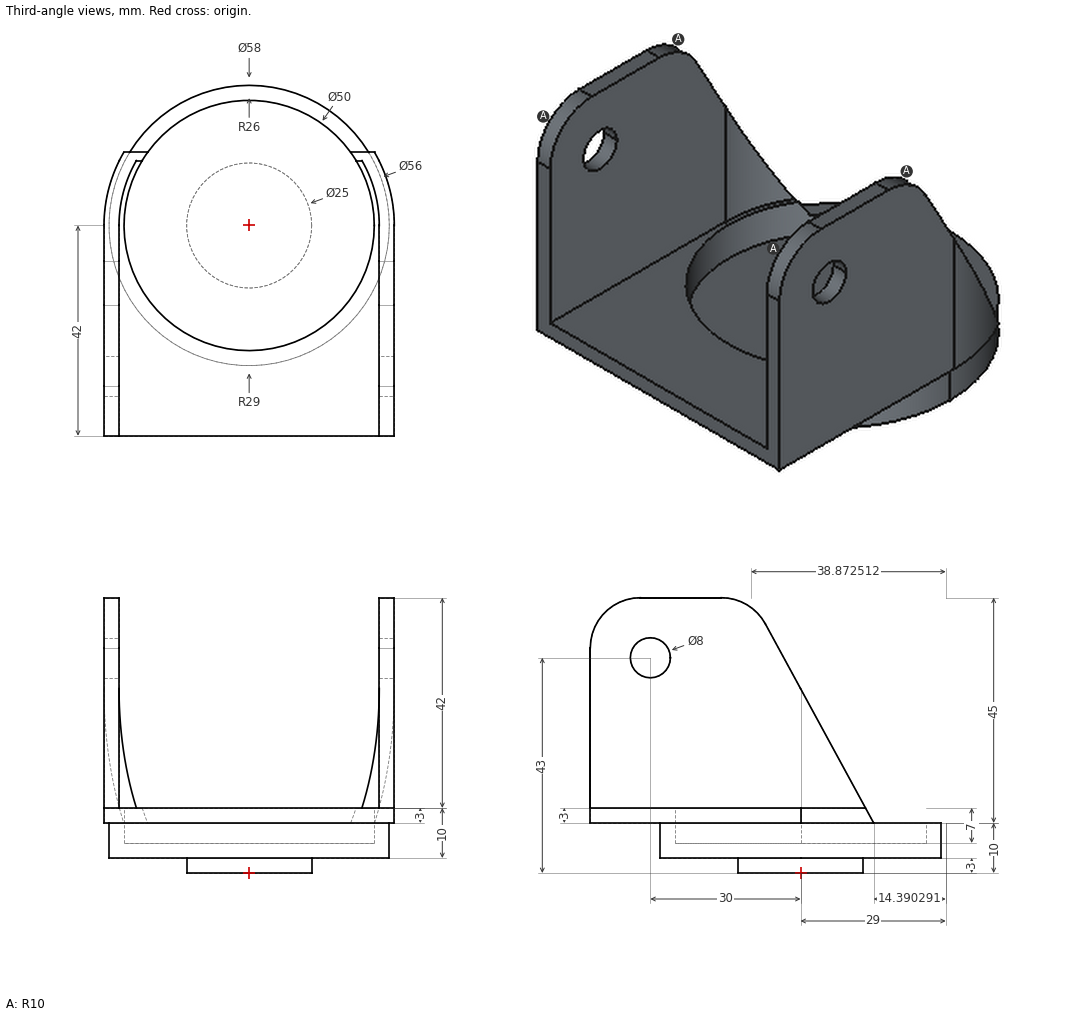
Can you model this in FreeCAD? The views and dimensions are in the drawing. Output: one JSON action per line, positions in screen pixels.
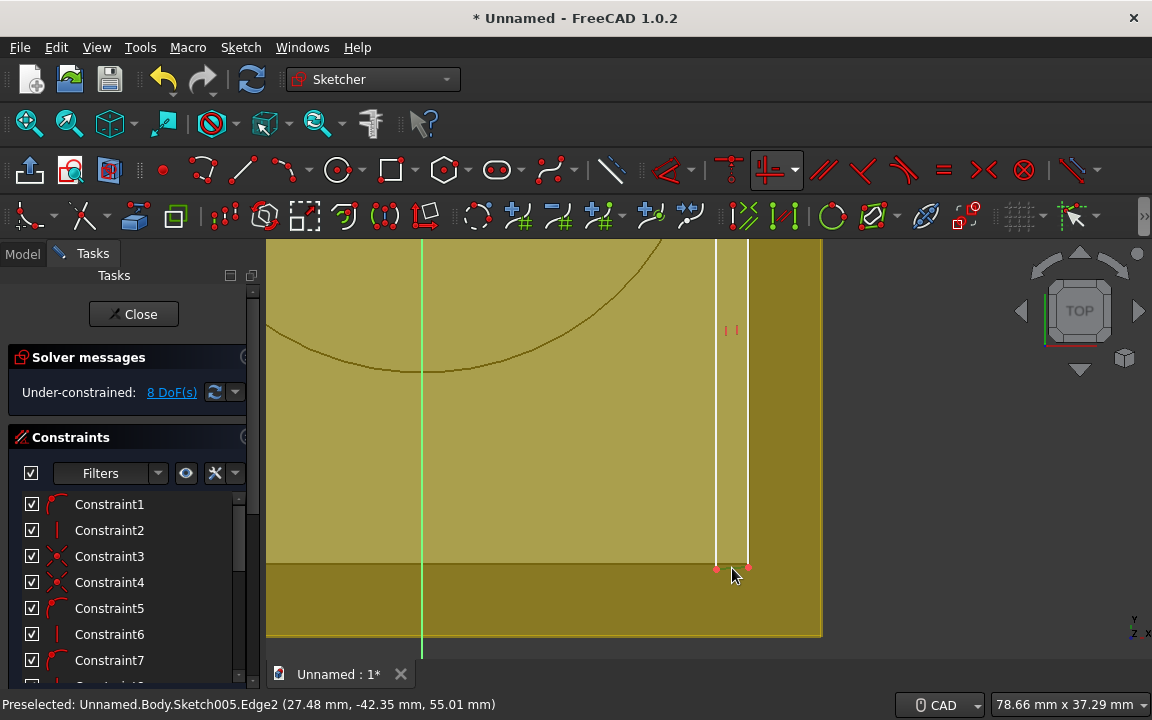
{"action": "key", "text": "h"}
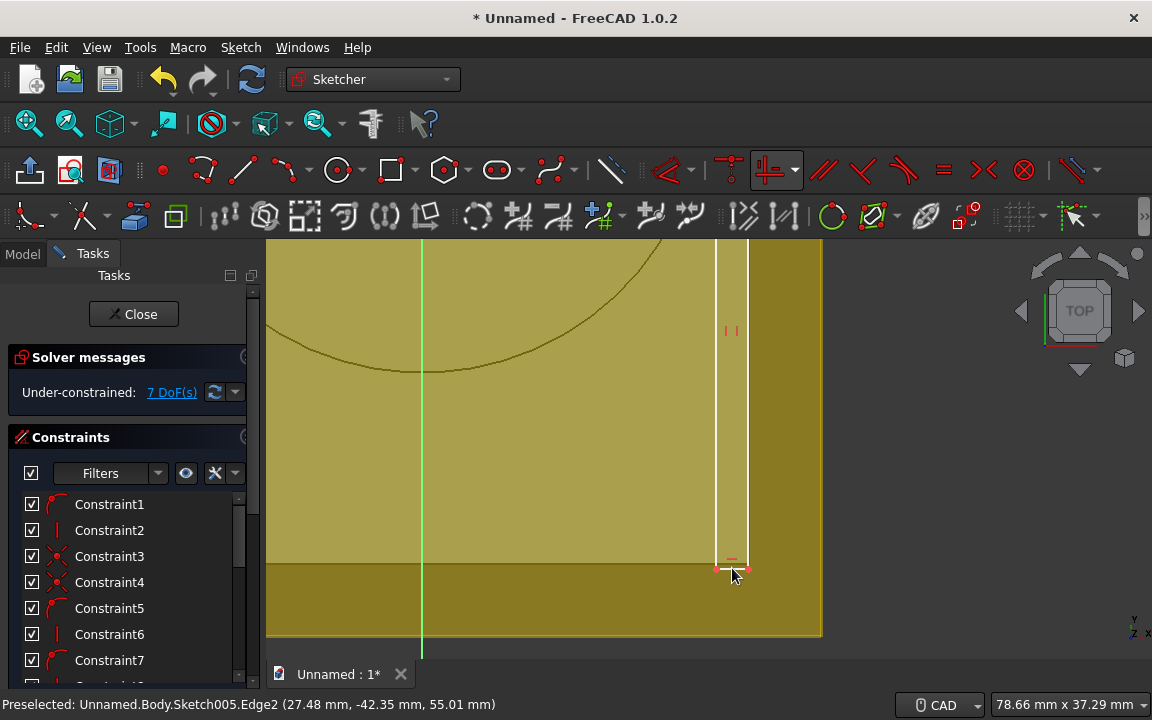
{"action": "scroll", "coordinate": [735, 572], "scroll_direction": "down", "scroll_amount": 6}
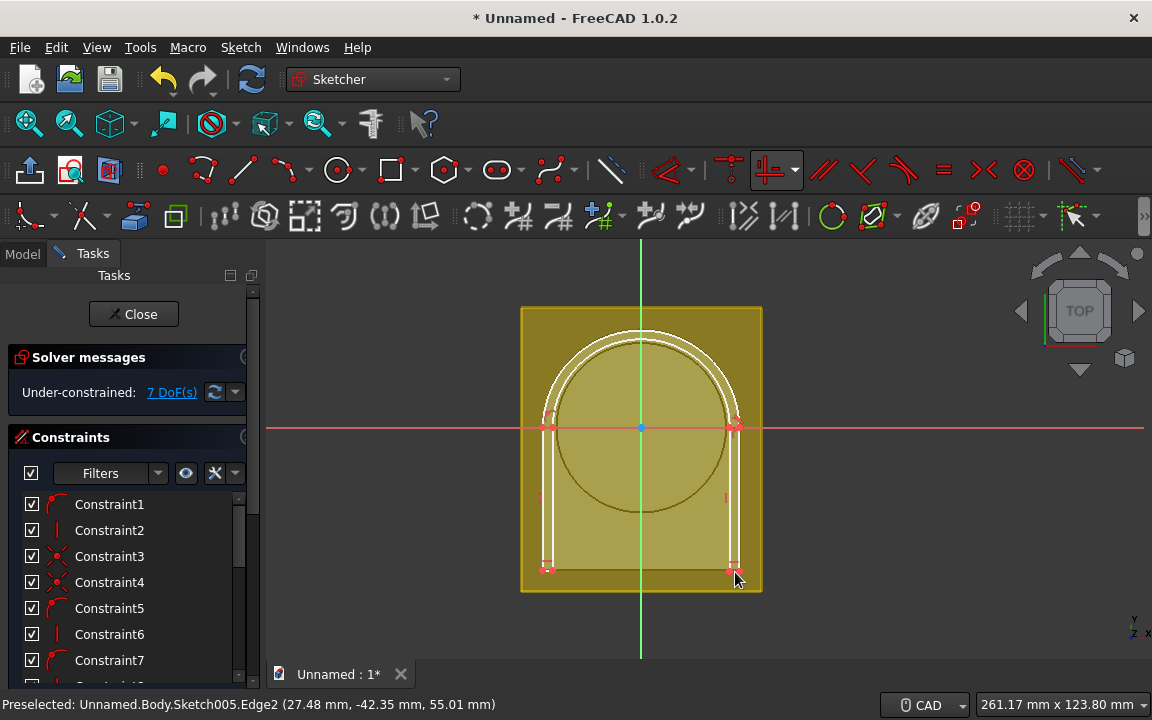
{"action": "scroll", "coordinate": [699, 349], "scroll_direction": "up", "scroll_amount": 3}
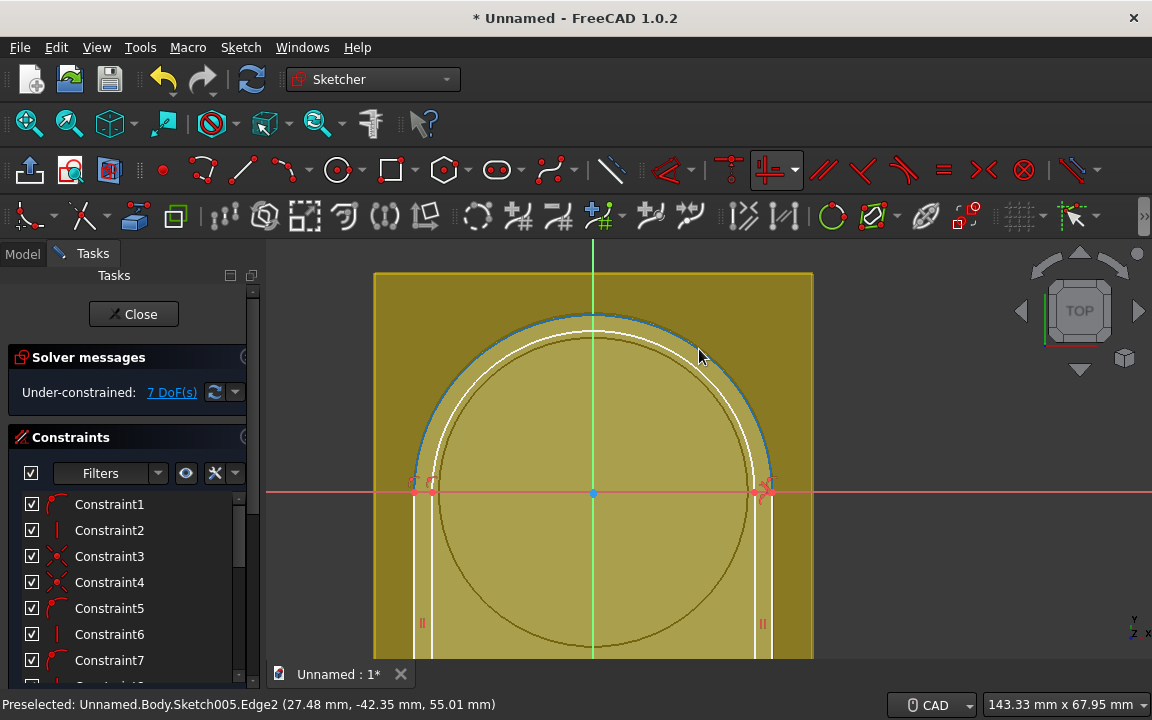
{"action": "left_click", "coordinate": [698, 349]}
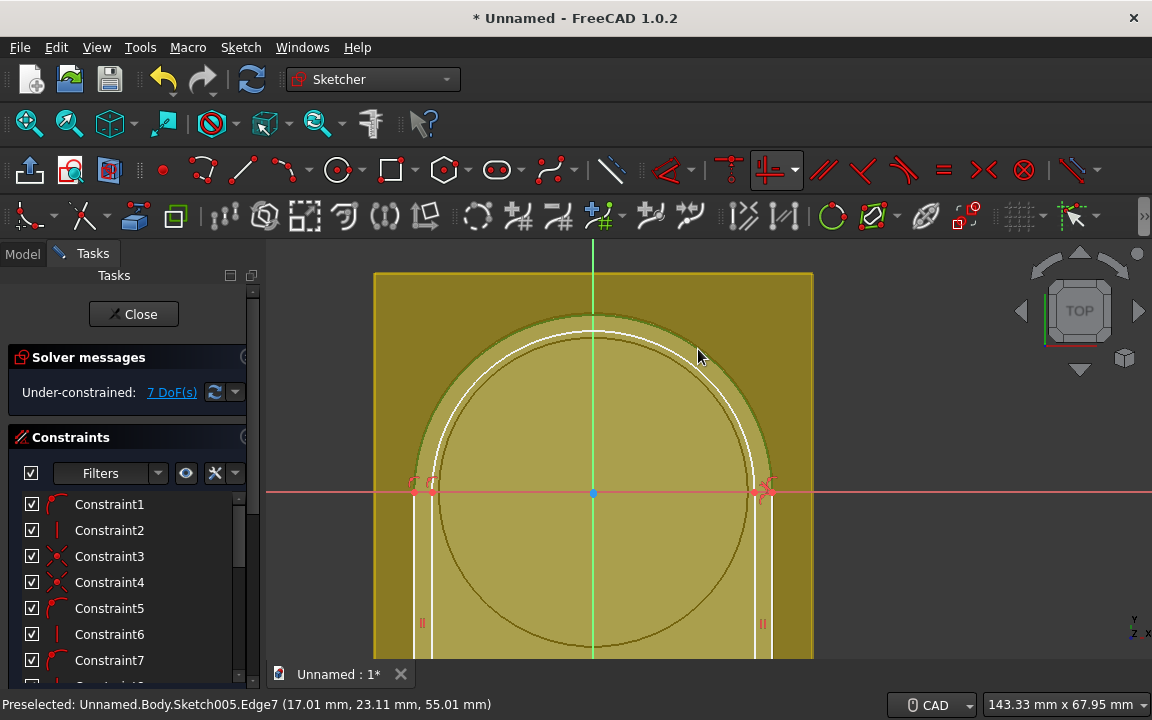
{"action": "left_click", "coordinate": [688, 362]}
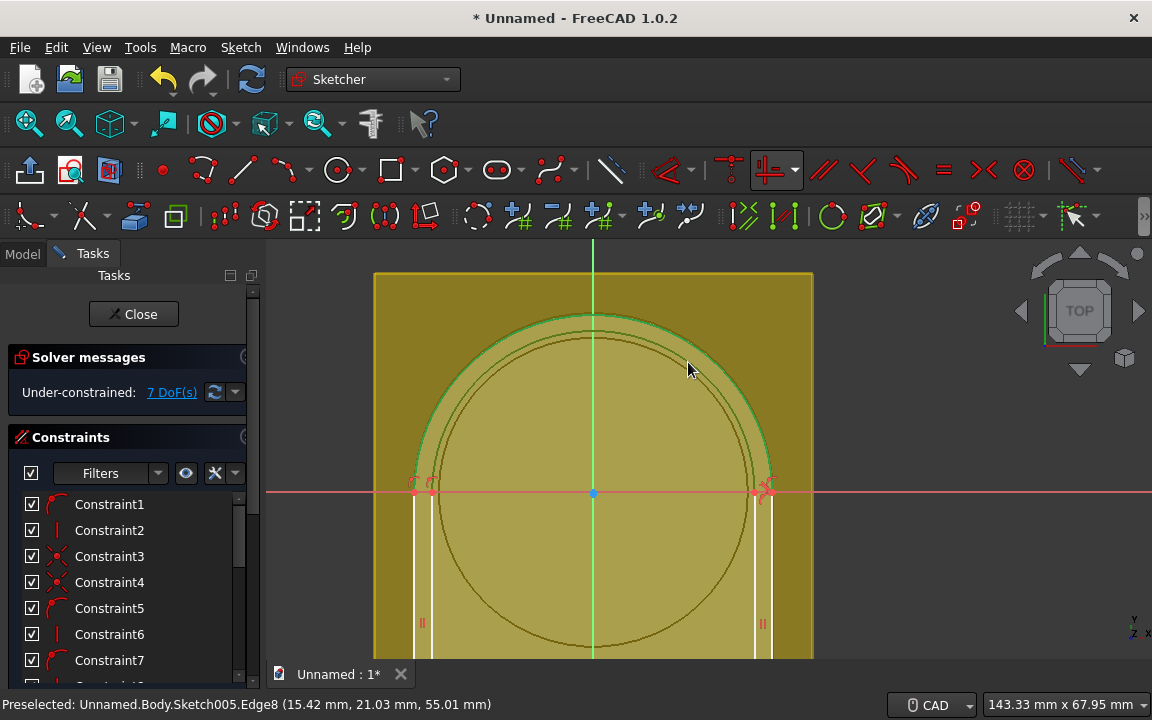
{"action": "left_click", "coordinate": [730, 170]}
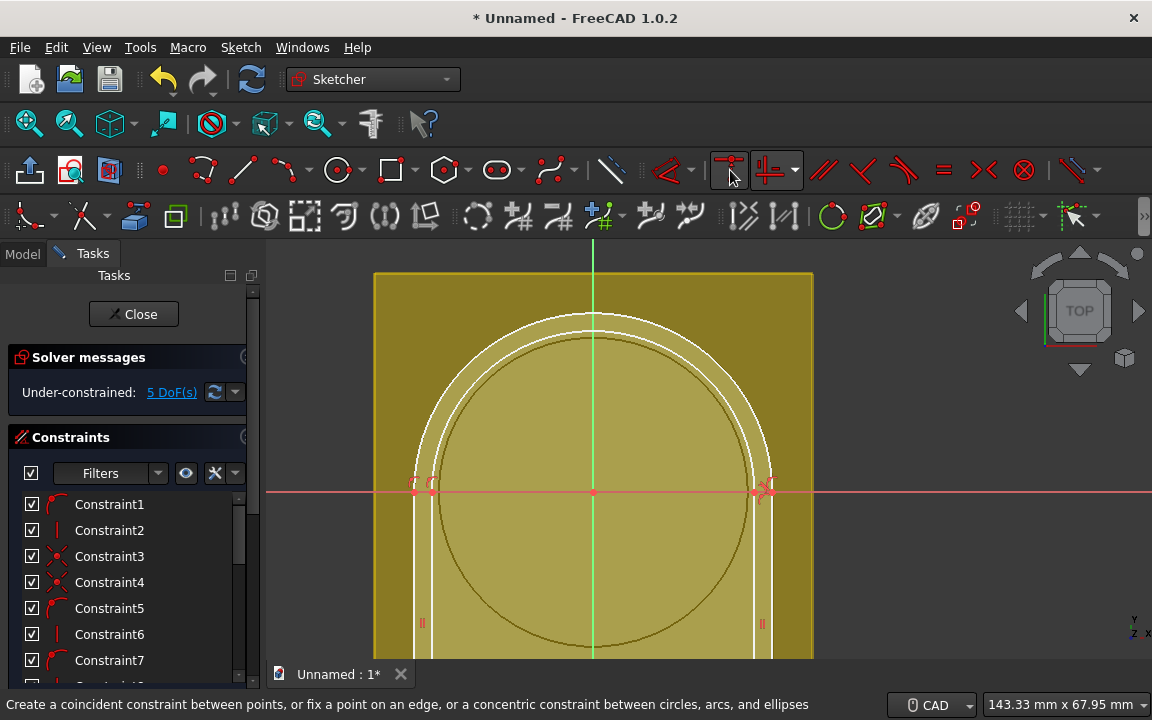
{"action": "left_click", "coordinate": [593, 492]}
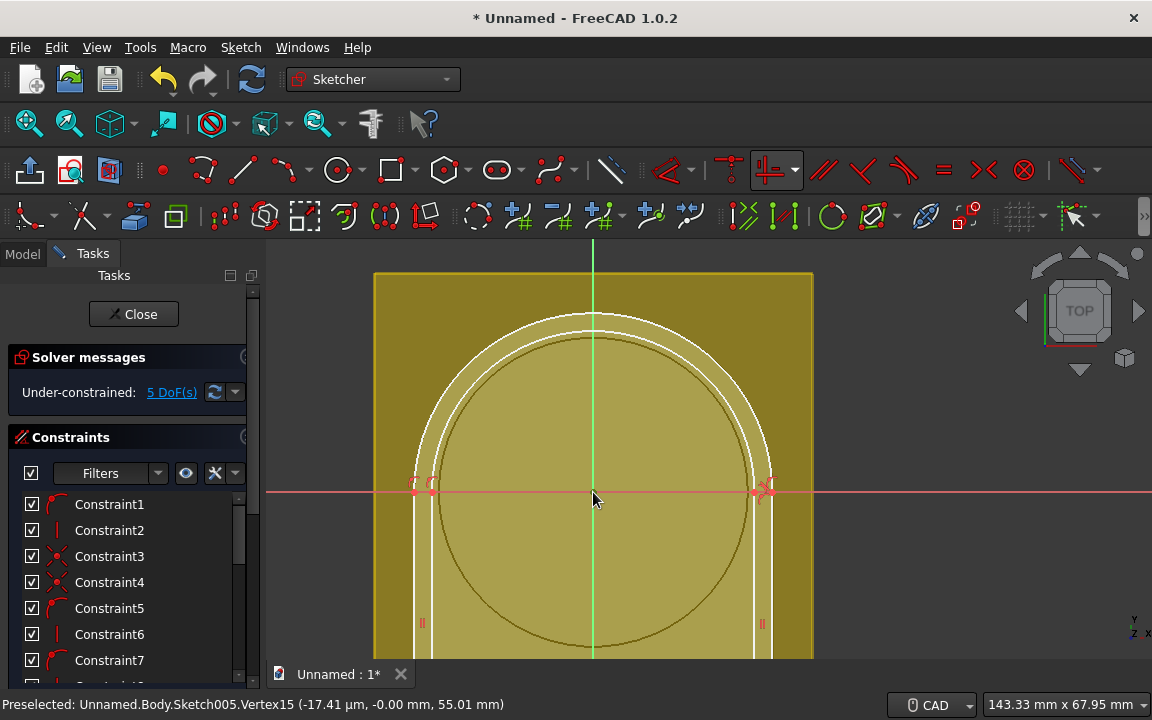
{"action": "left_click", "coordinate": [593, 605]}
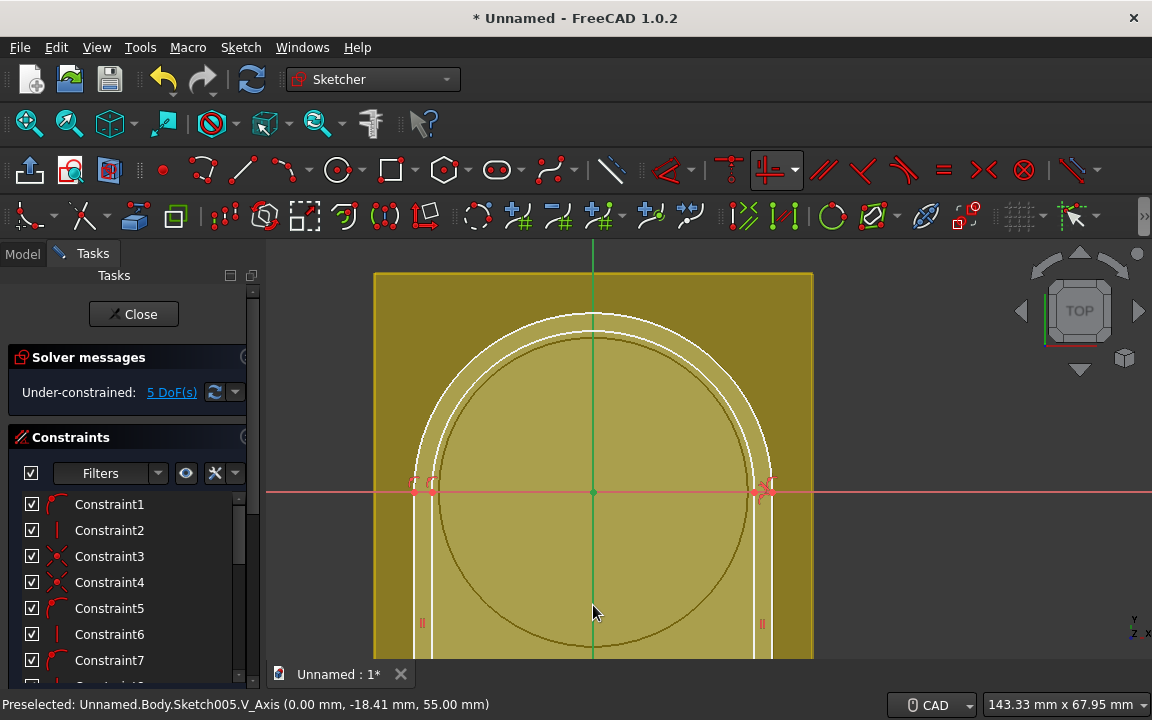
{"action": "left_click", "coordinate": [730, 170]}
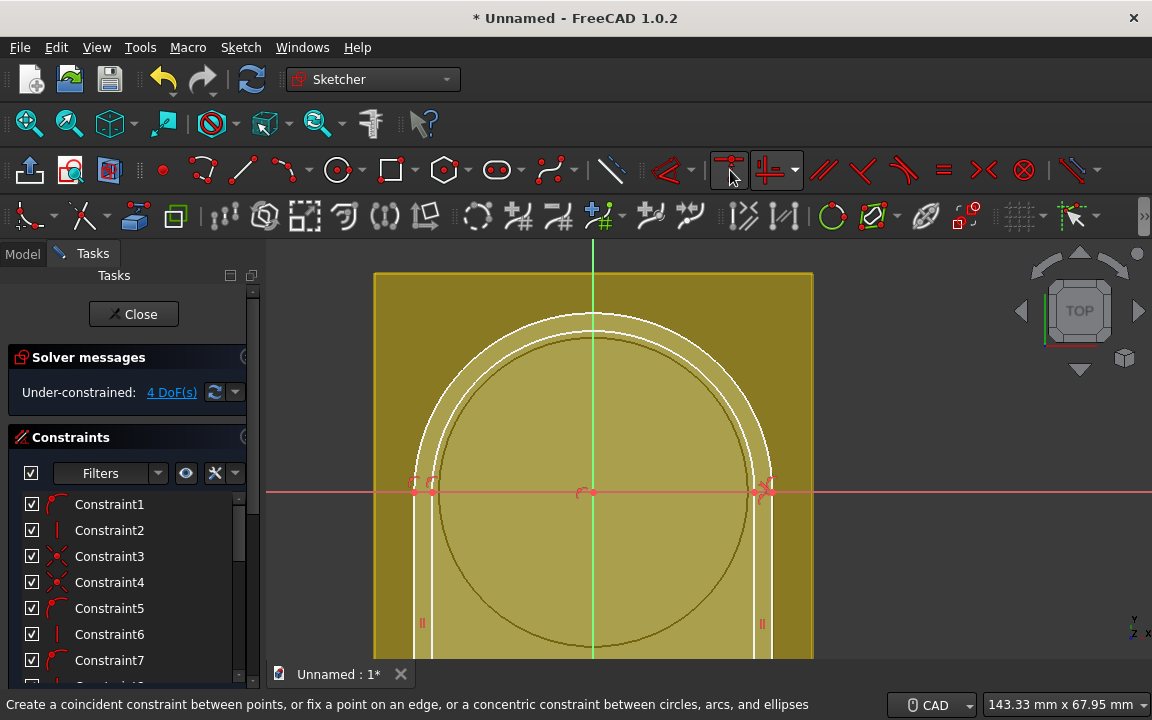
{"action": "left_click", "coordinate": [666, 170]}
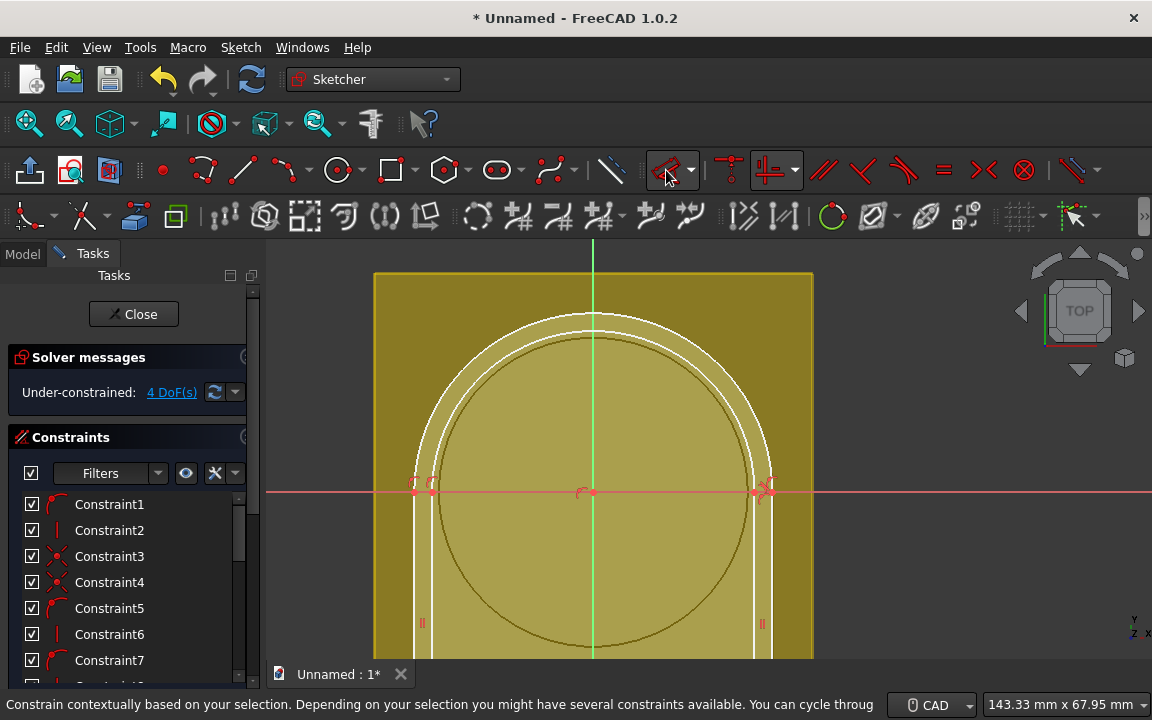
{"action": "left_click", "coordinate": [699, 347]}
{"action": "left_click", "coordinate": [718, 321]}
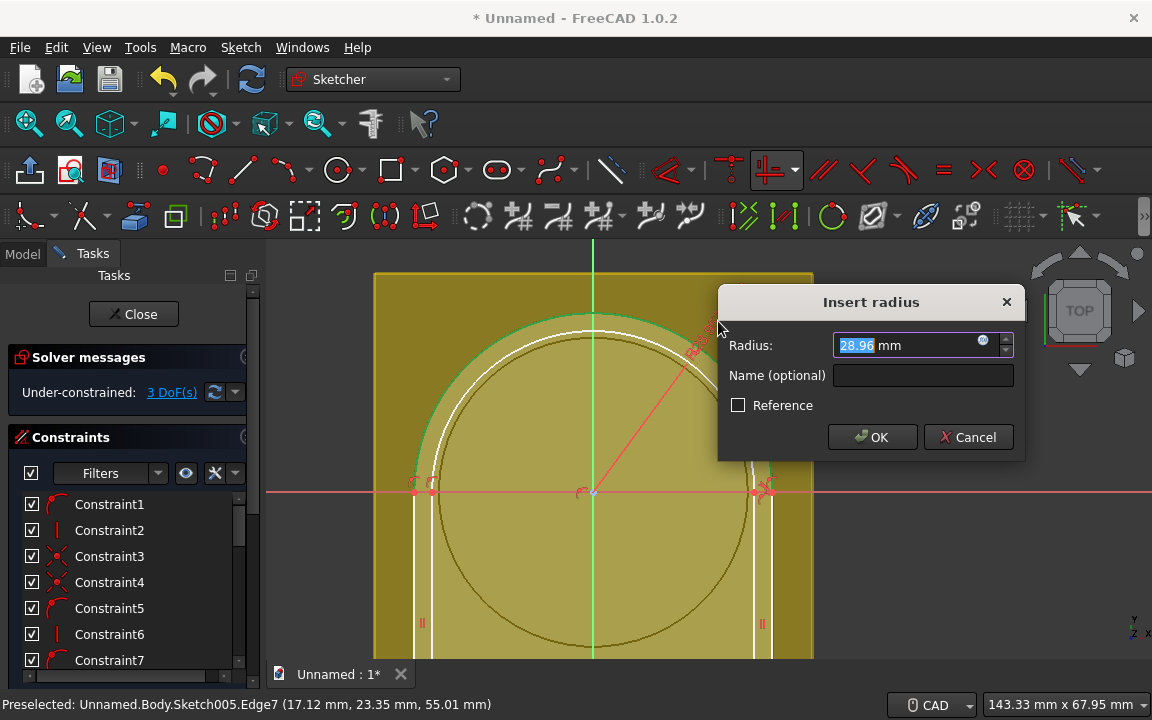
{"action": "type", "text": "29"}
{"action": "key", "text": "Return"}